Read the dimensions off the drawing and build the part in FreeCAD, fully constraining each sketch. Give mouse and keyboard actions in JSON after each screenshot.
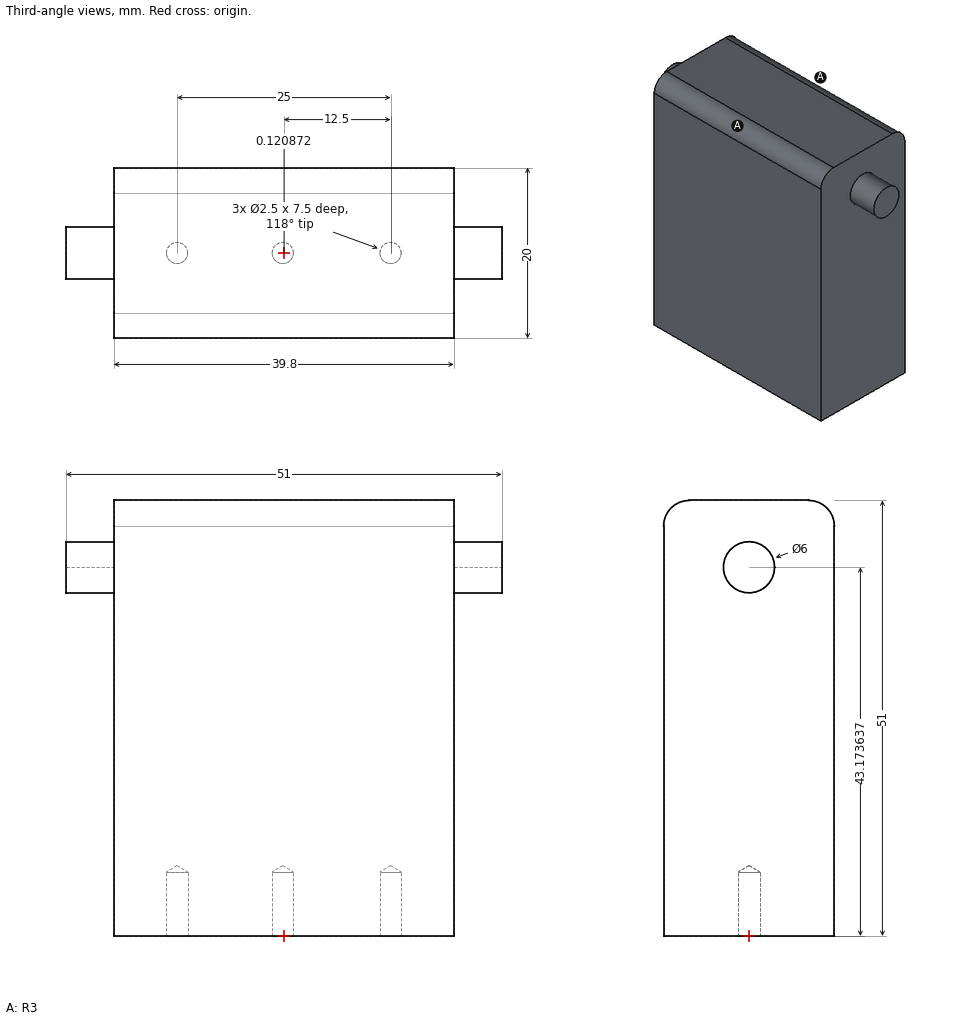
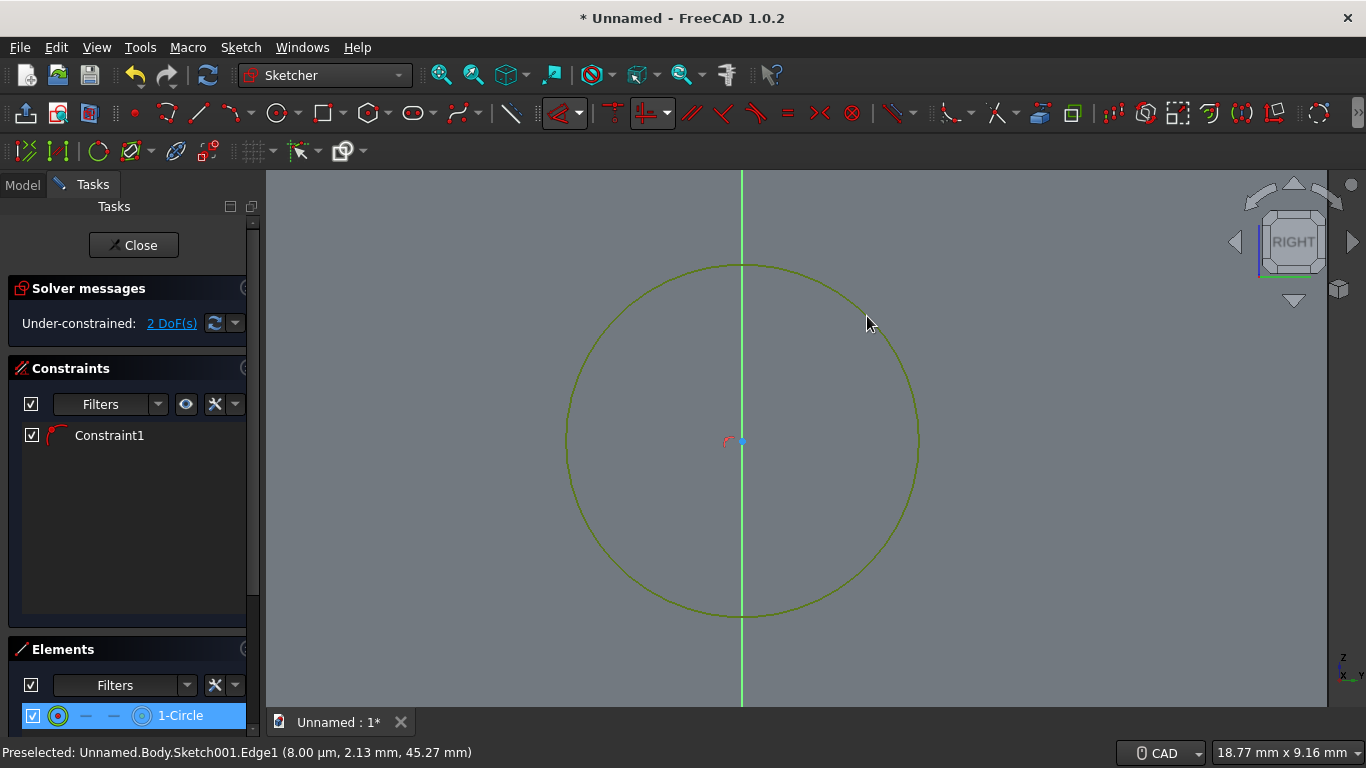
{"action": "key", "text": "k o"}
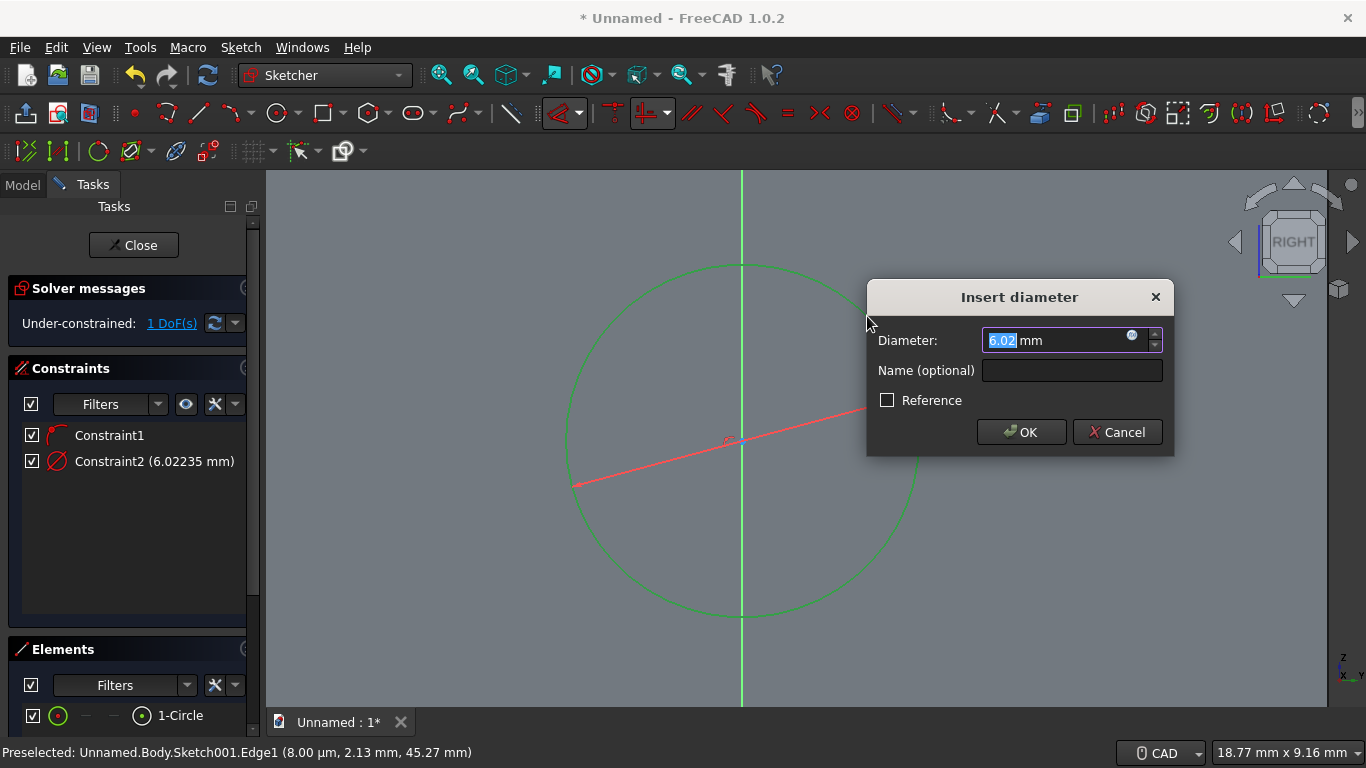
{"action": "type", "text": "6"}
{"action": "key", "text": "Return"}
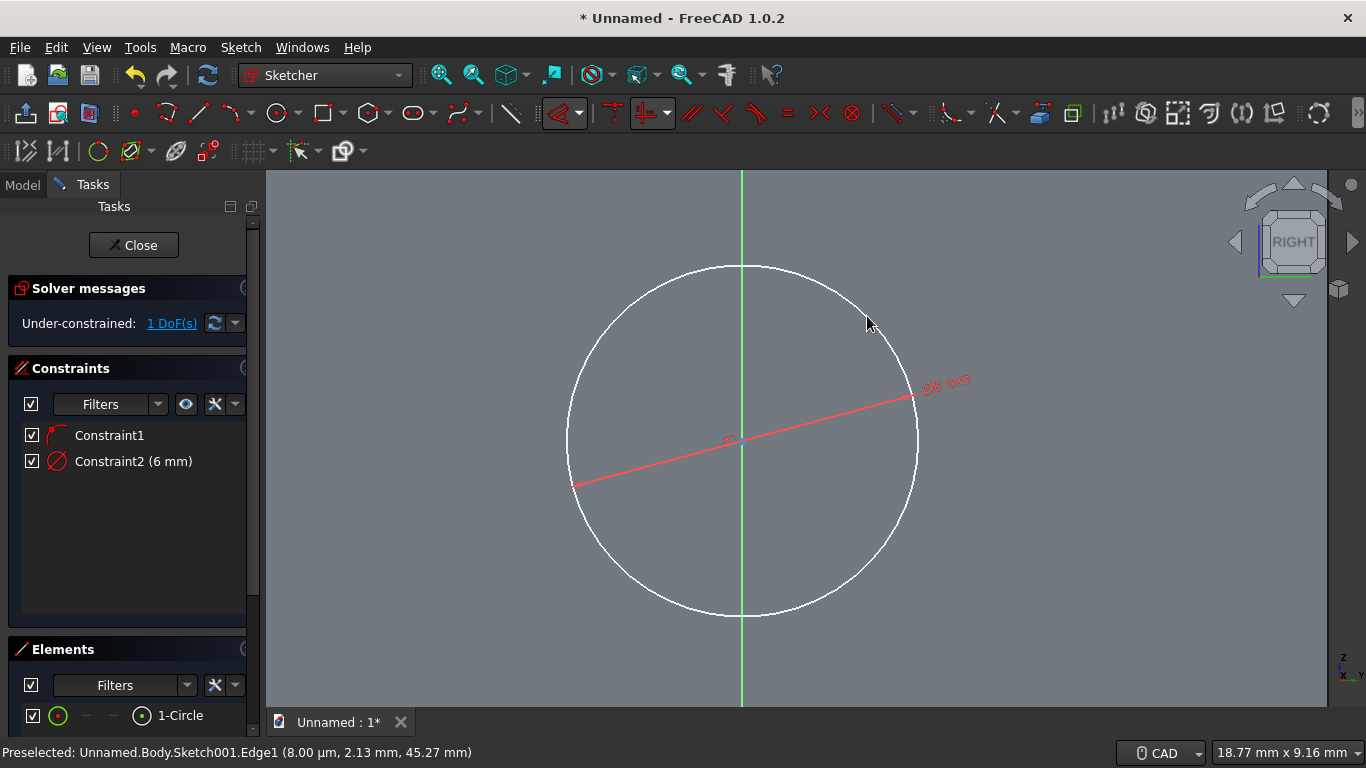
{"action": "left_click", "coordinate": [742, 441]}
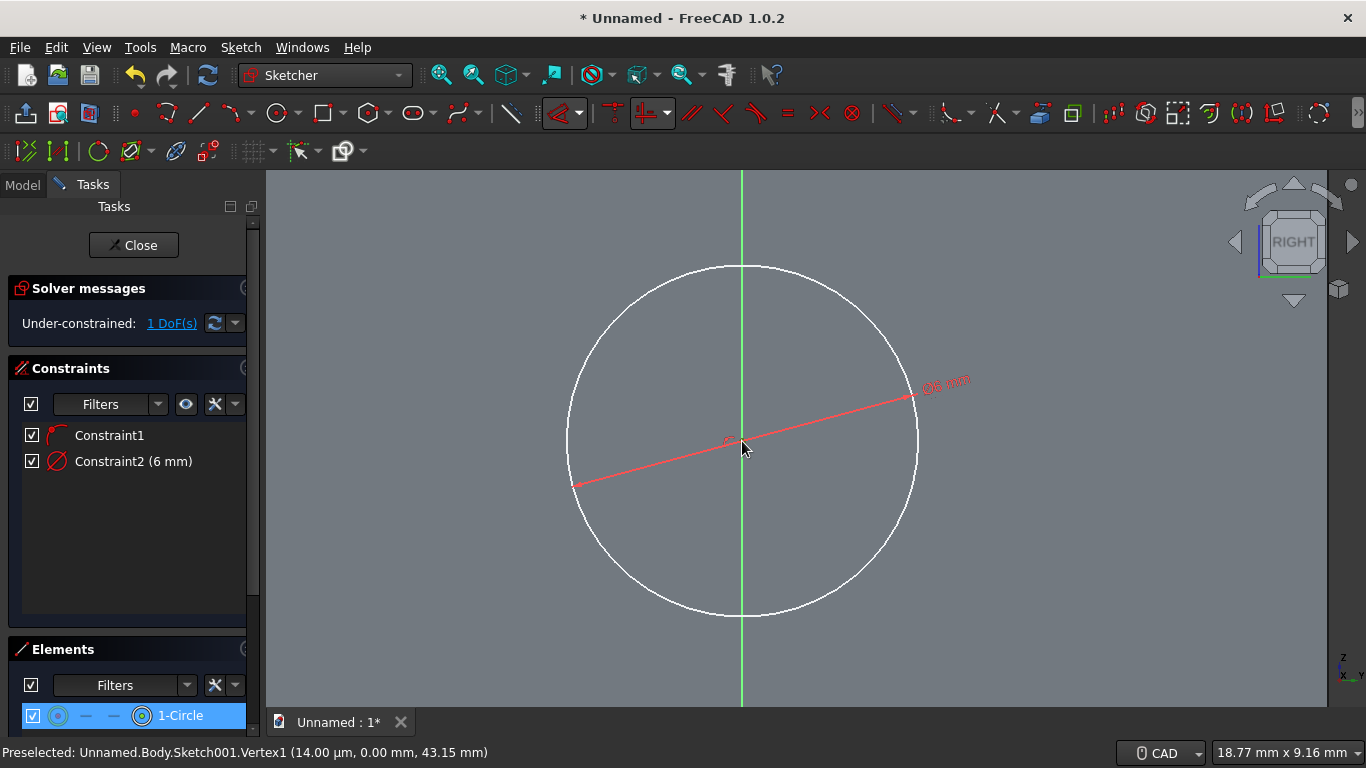
{"action": "key", "text": "i"}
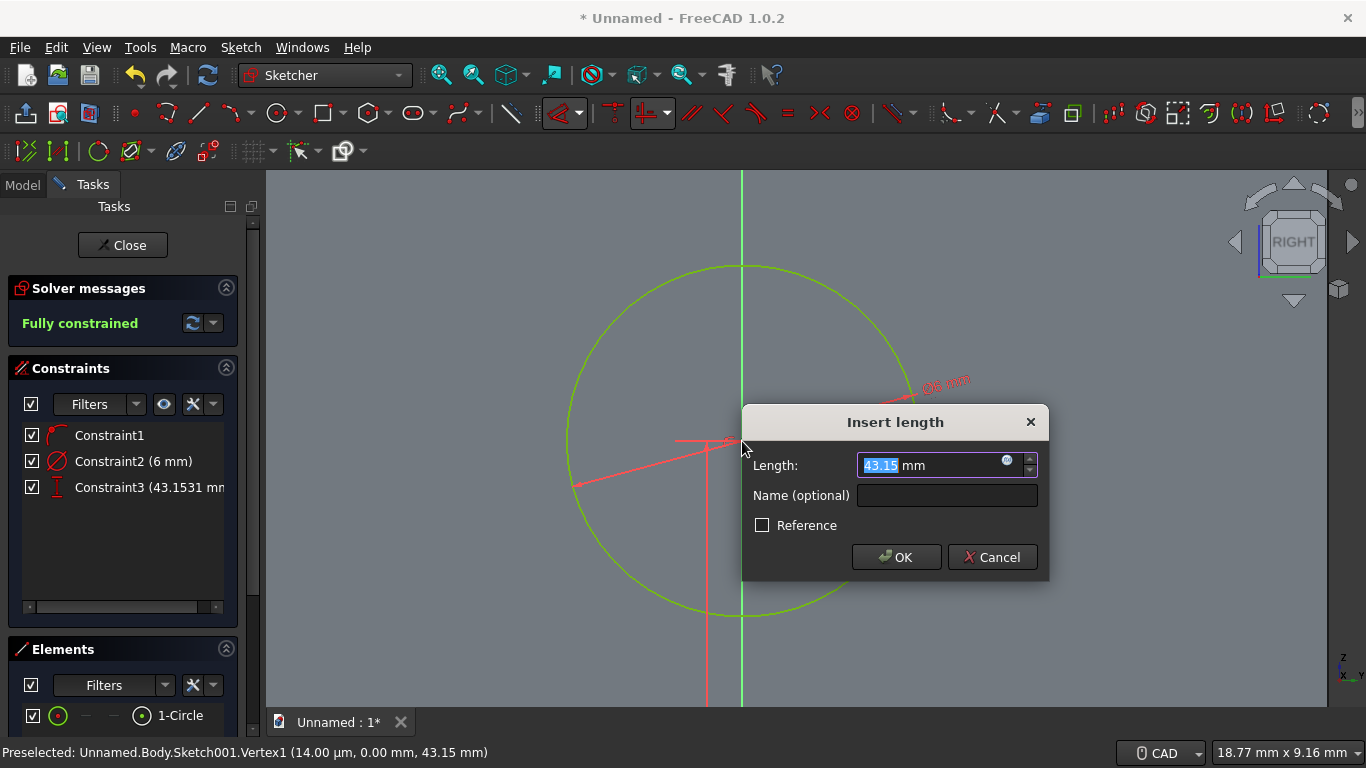
{"action": "type", "text": "43.173637"}
{"action": "key", "text": "Return"}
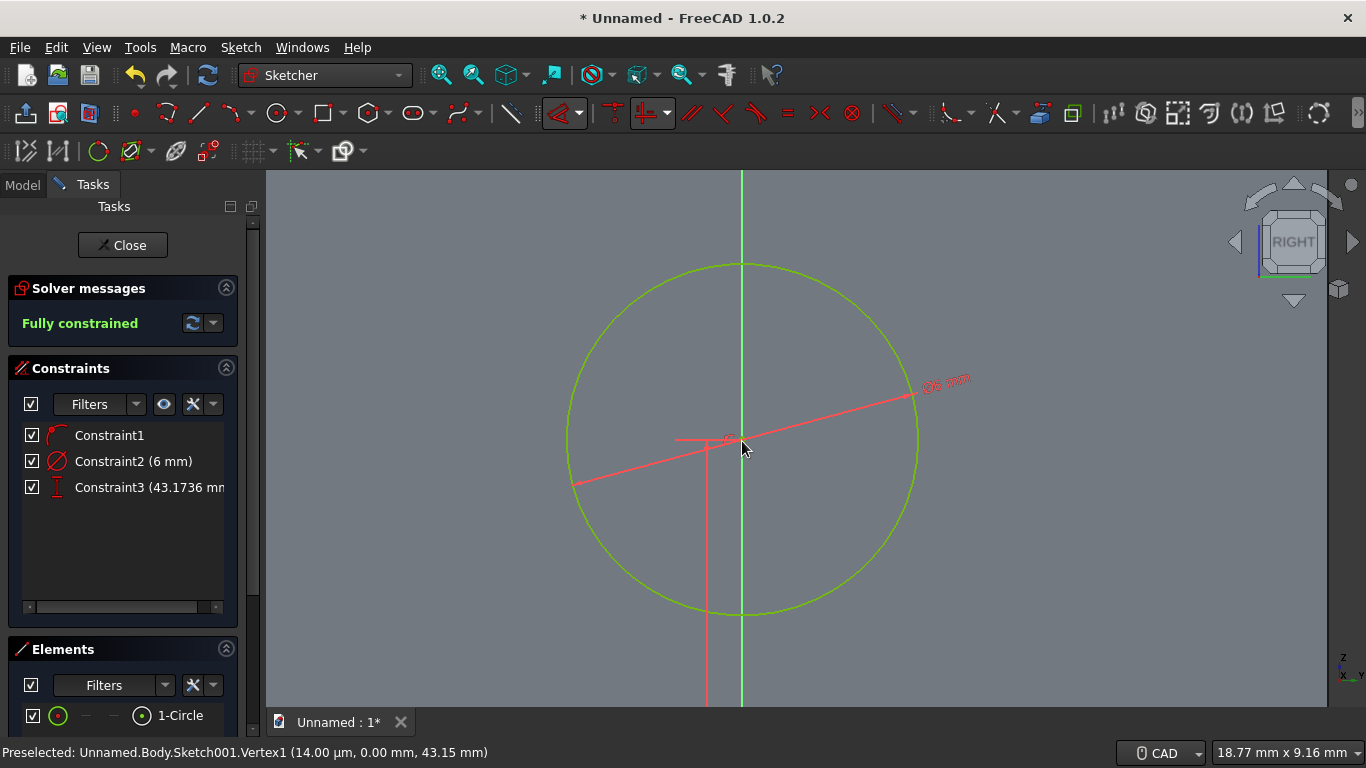
{"action": "left_click", "coordinate": [123, 245]}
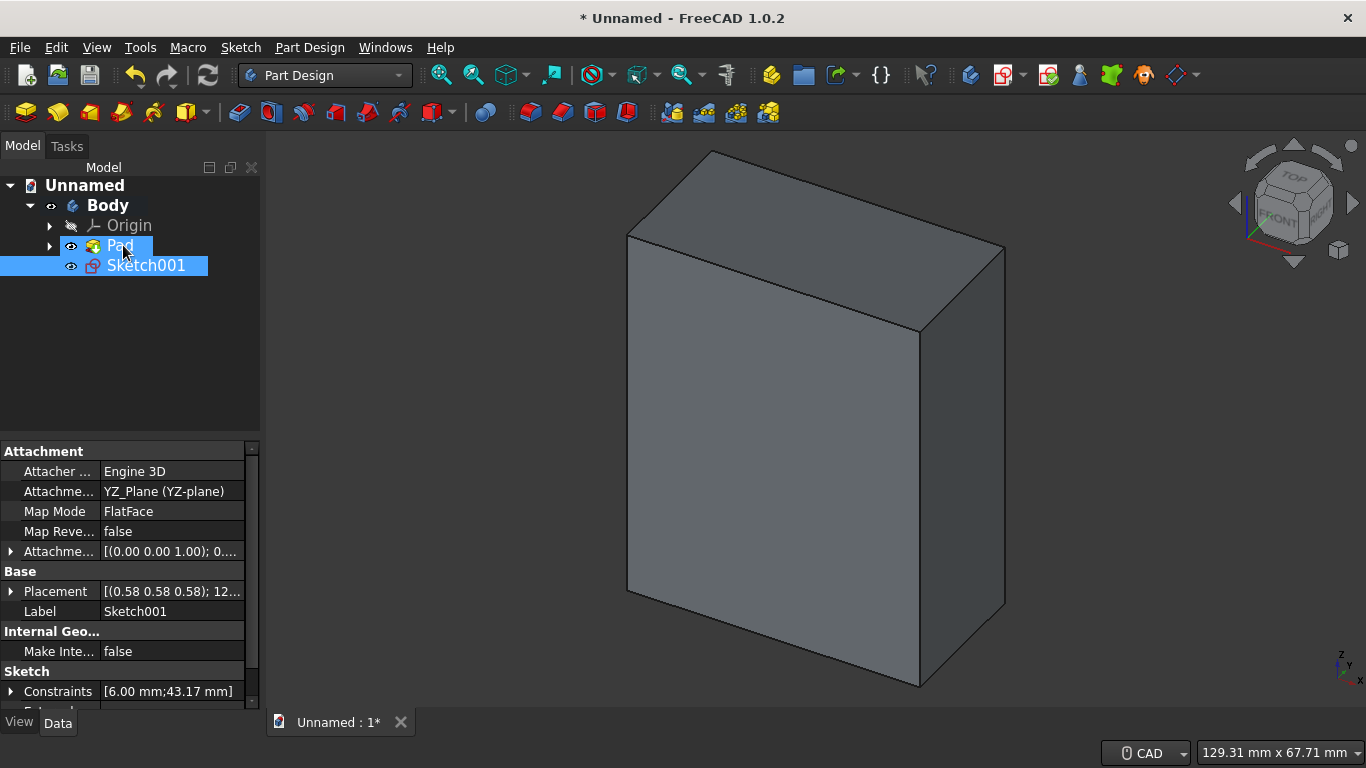
{"action": "left_click", "coordinate": [26, 112]}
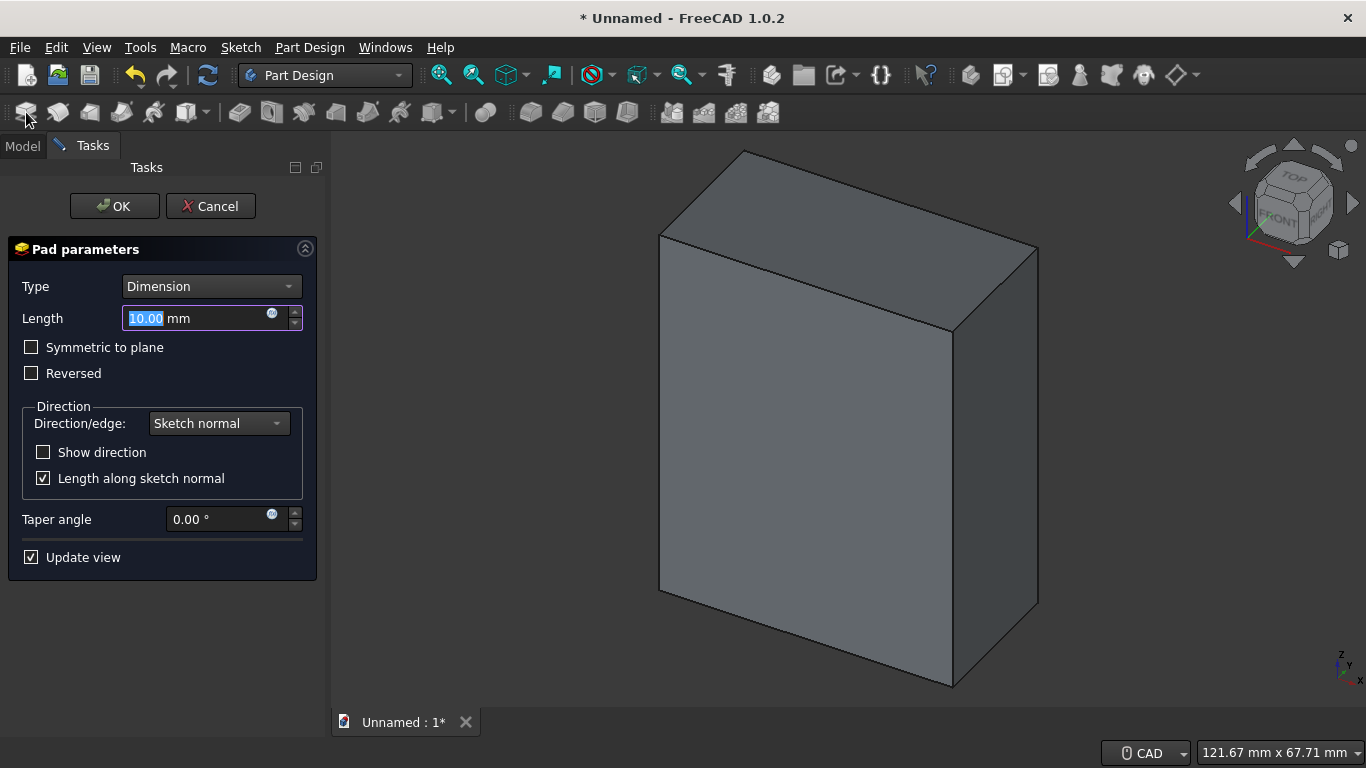
{"action": "type", "text": "51"}
{"action": "key", "text": "Tab"}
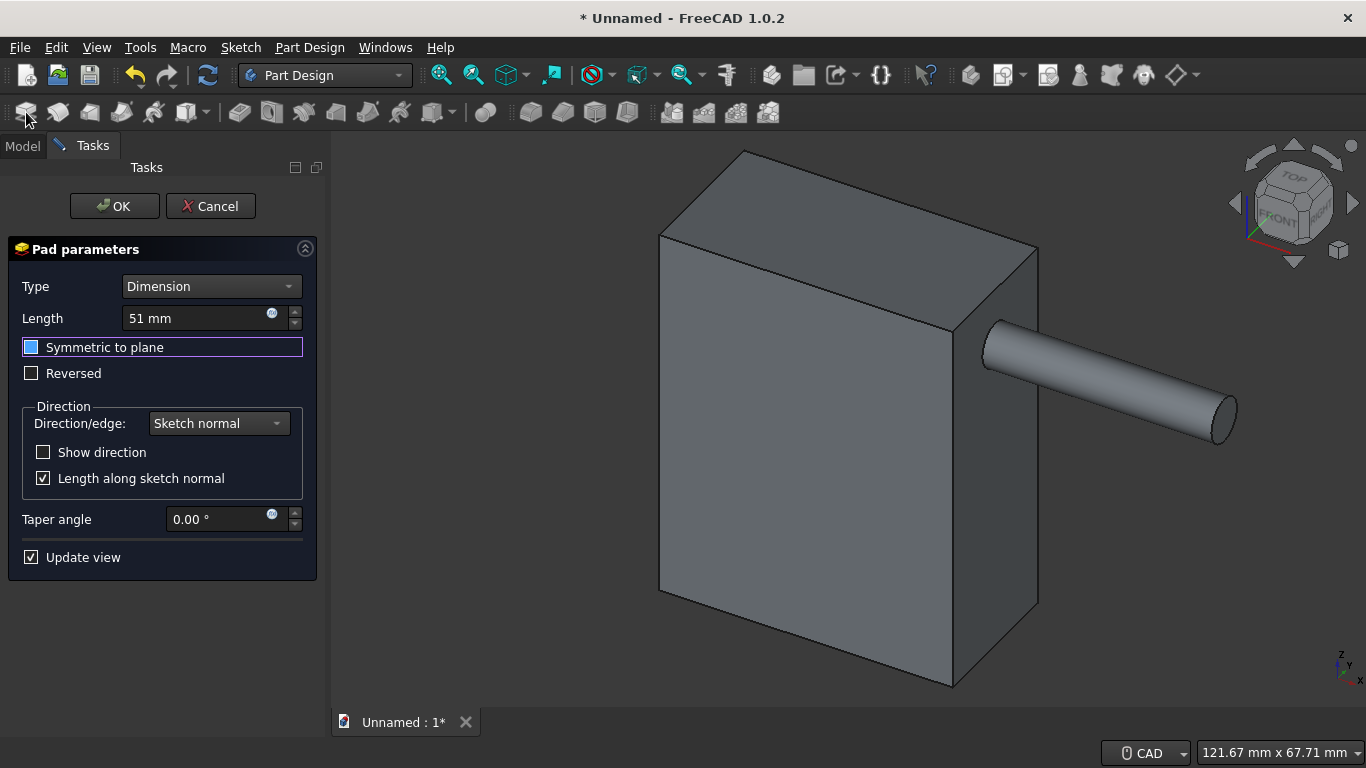
{"action": "left_click", "coordinate": [30, 347]}